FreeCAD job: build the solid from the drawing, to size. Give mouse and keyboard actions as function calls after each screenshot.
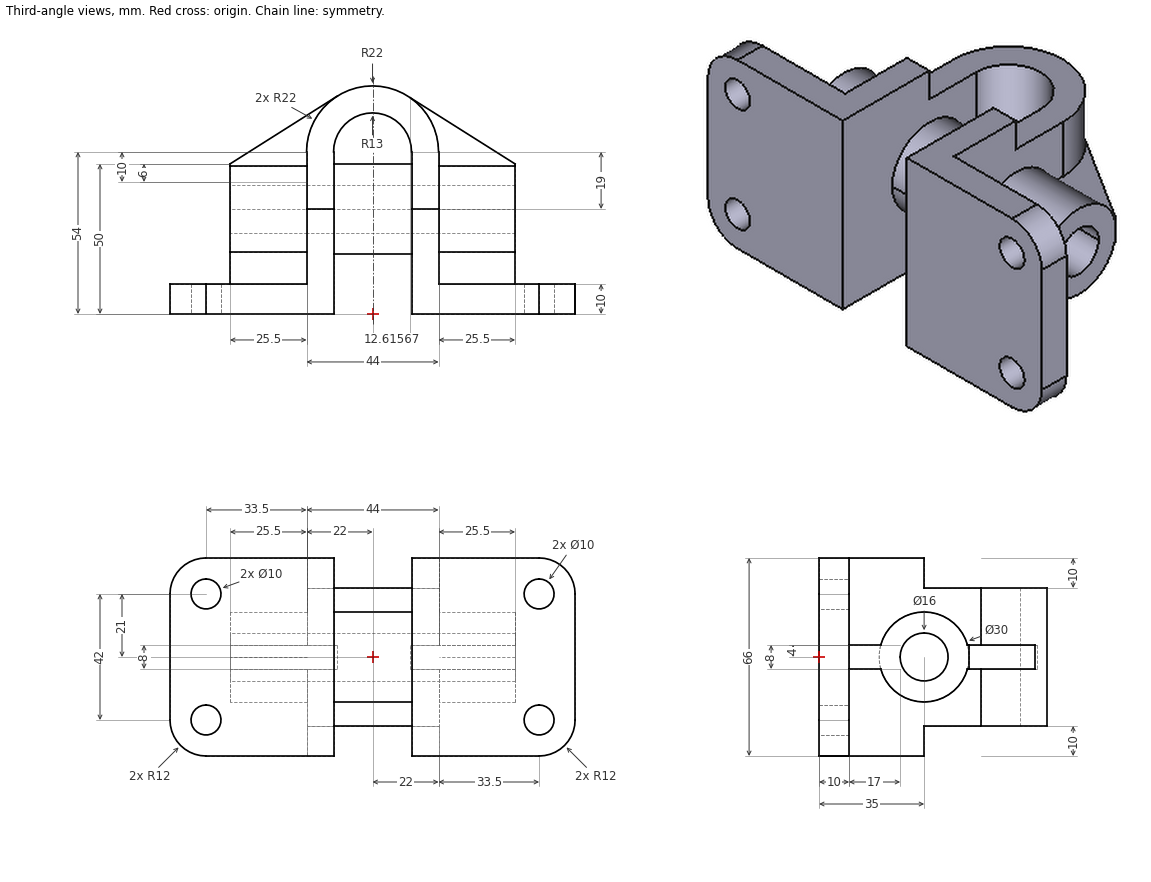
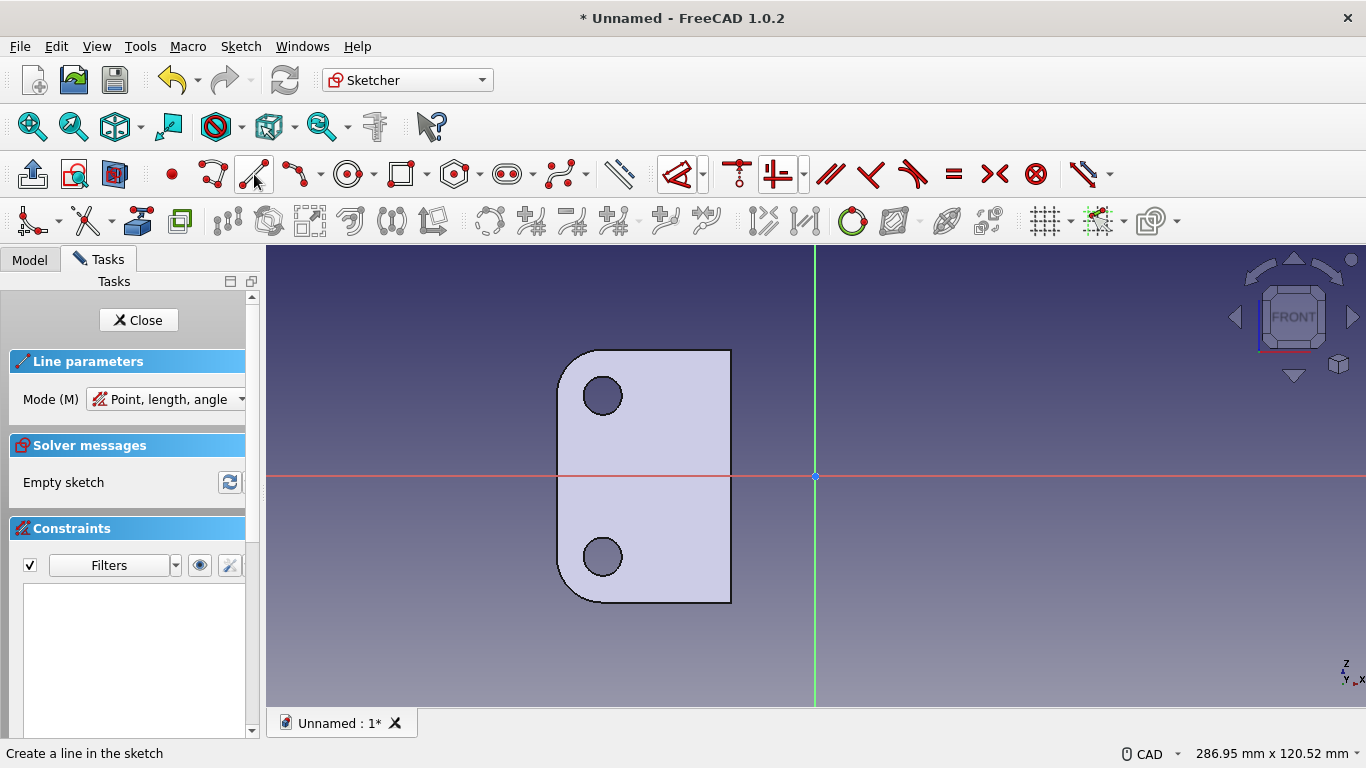
click(1074, 396)
click(1074, 557)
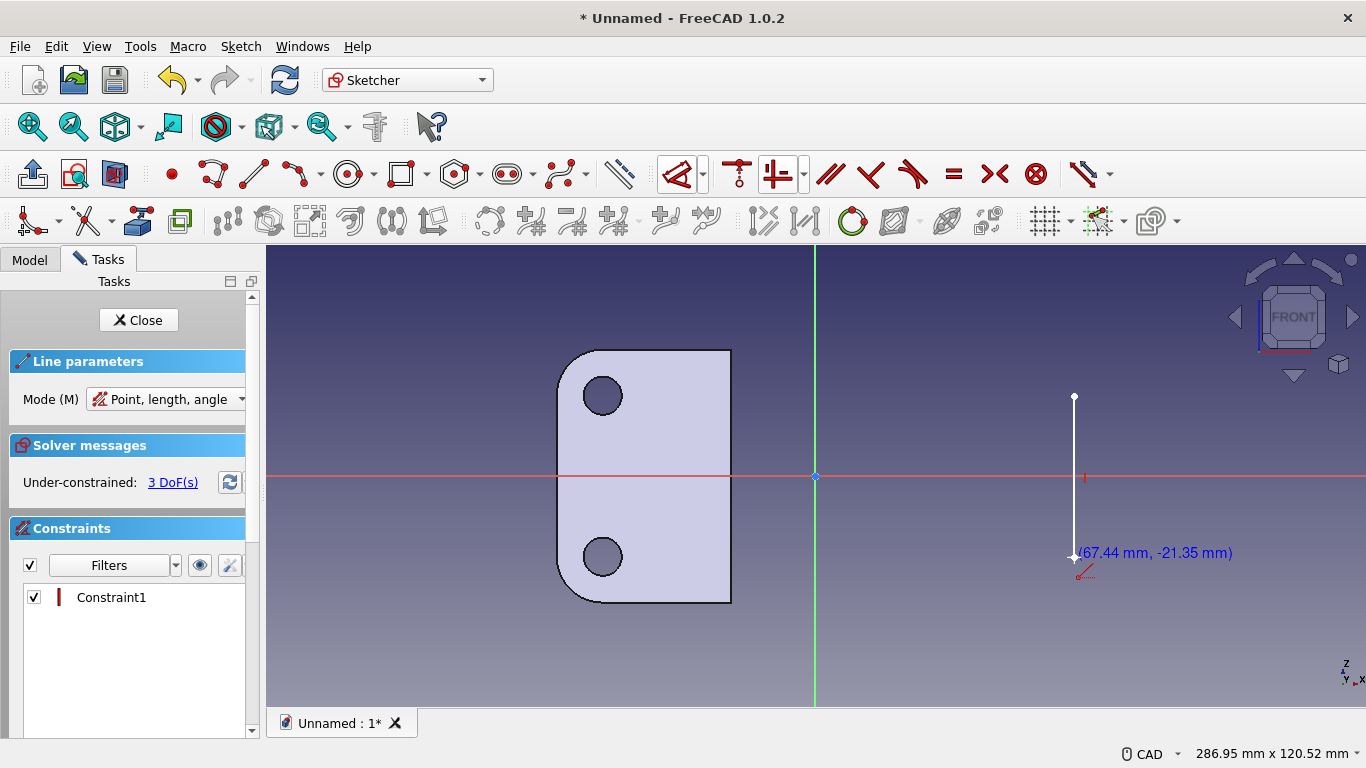
click(213, 174)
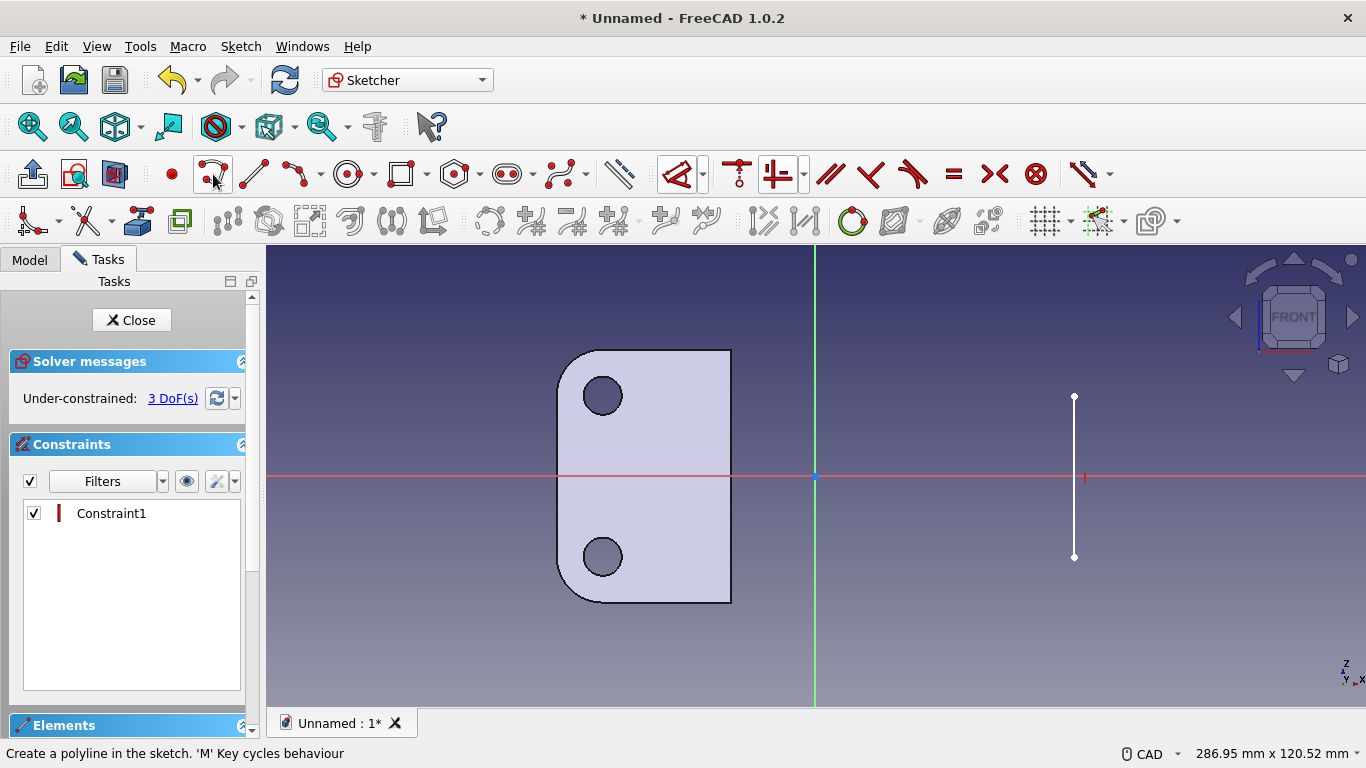
click(1028, 603)
click(900, 603)
click(900, 350)
click(1028, 350)
right_click(1028, 350)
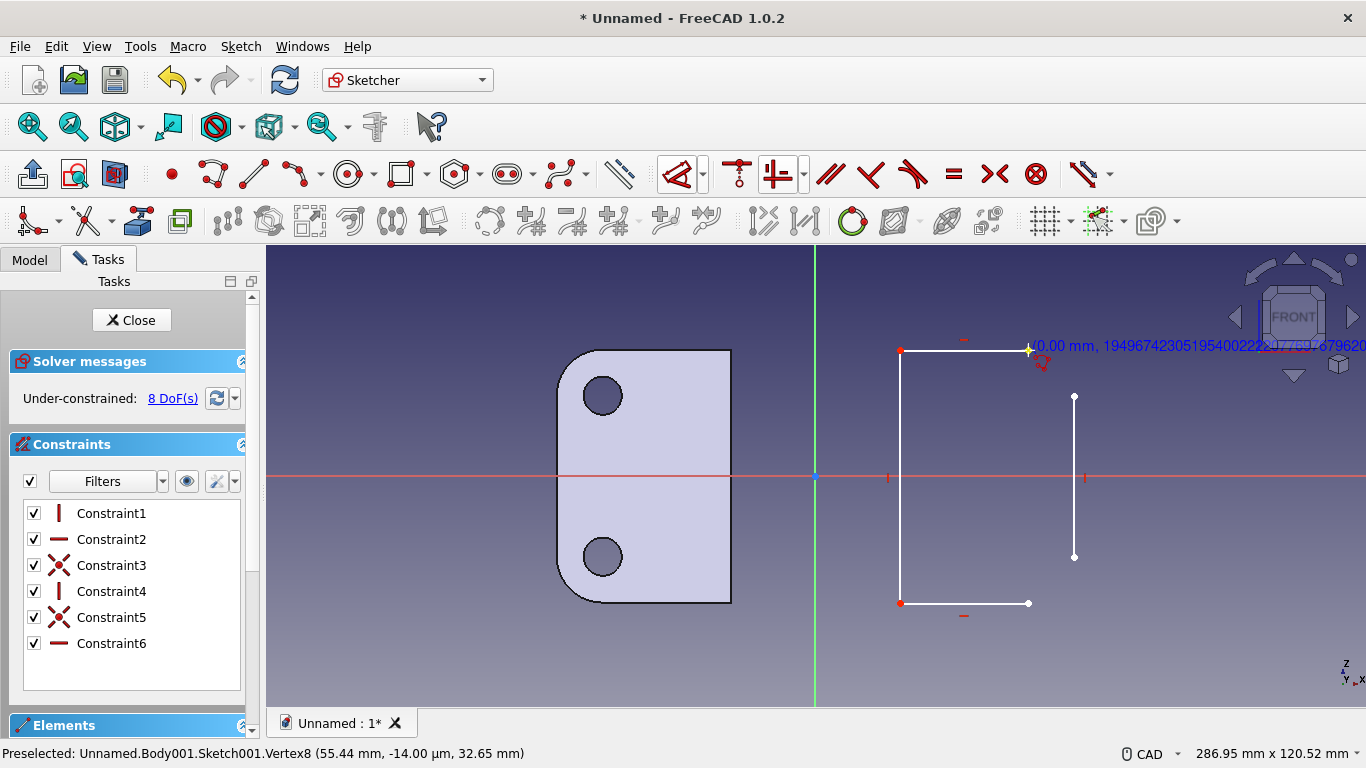
click(294, 174)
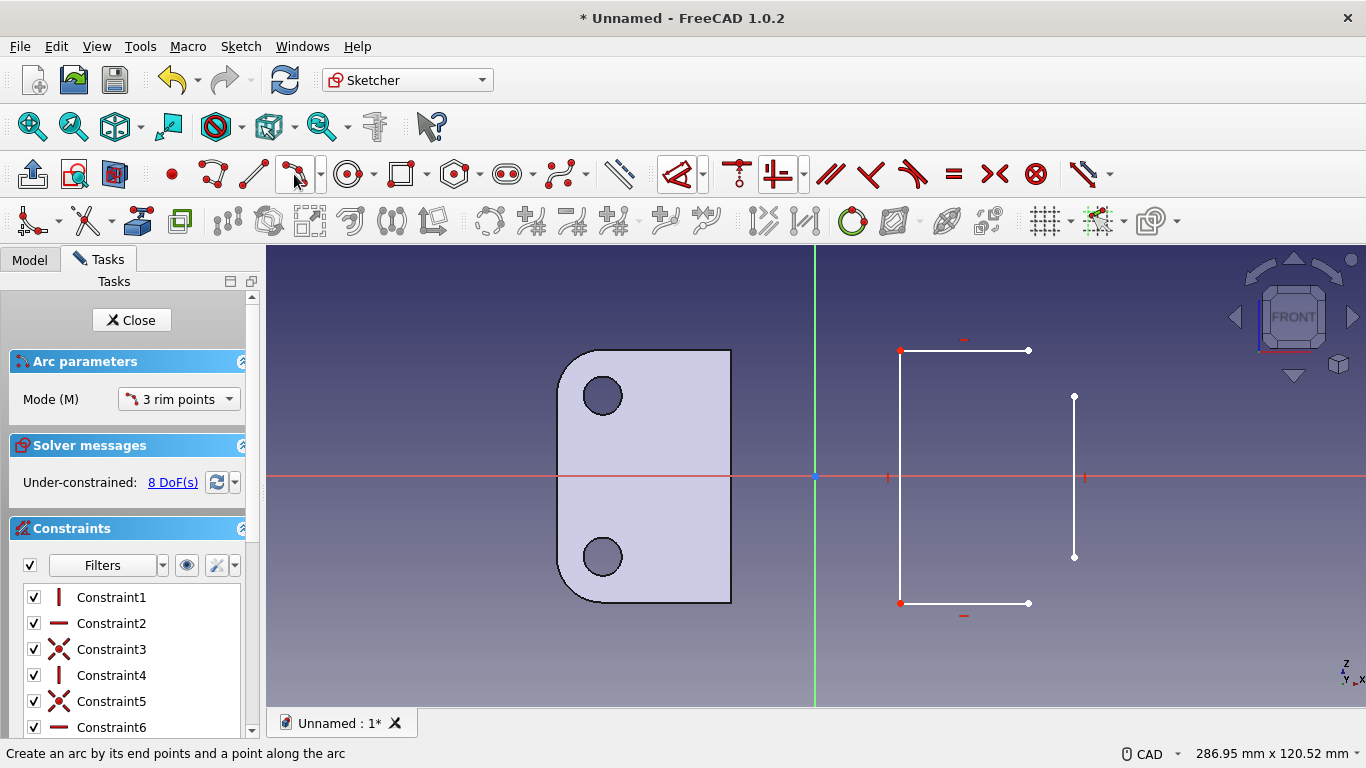
click(1074, 558)
click(1028, 604)
click(1061, 589)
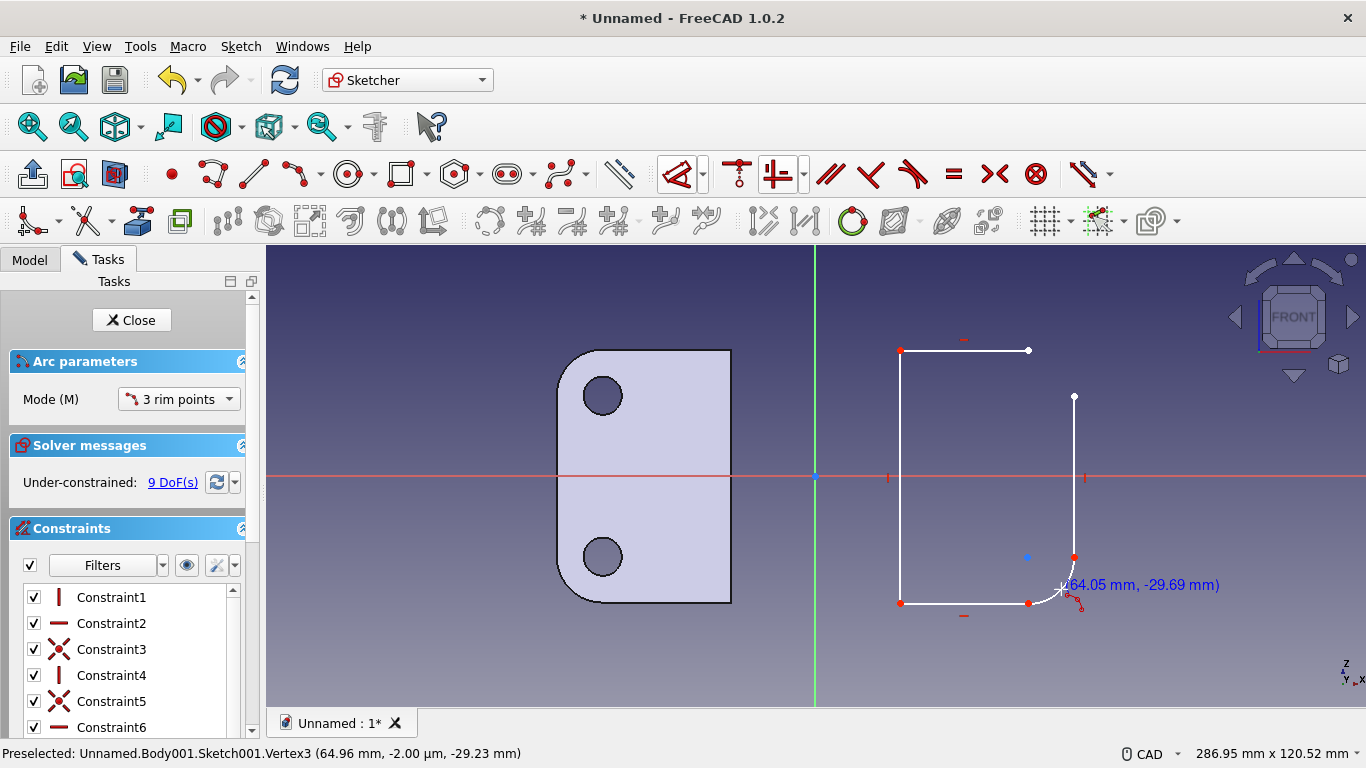
click(1028, 351)
click(1074, 397)
click(1061, 363)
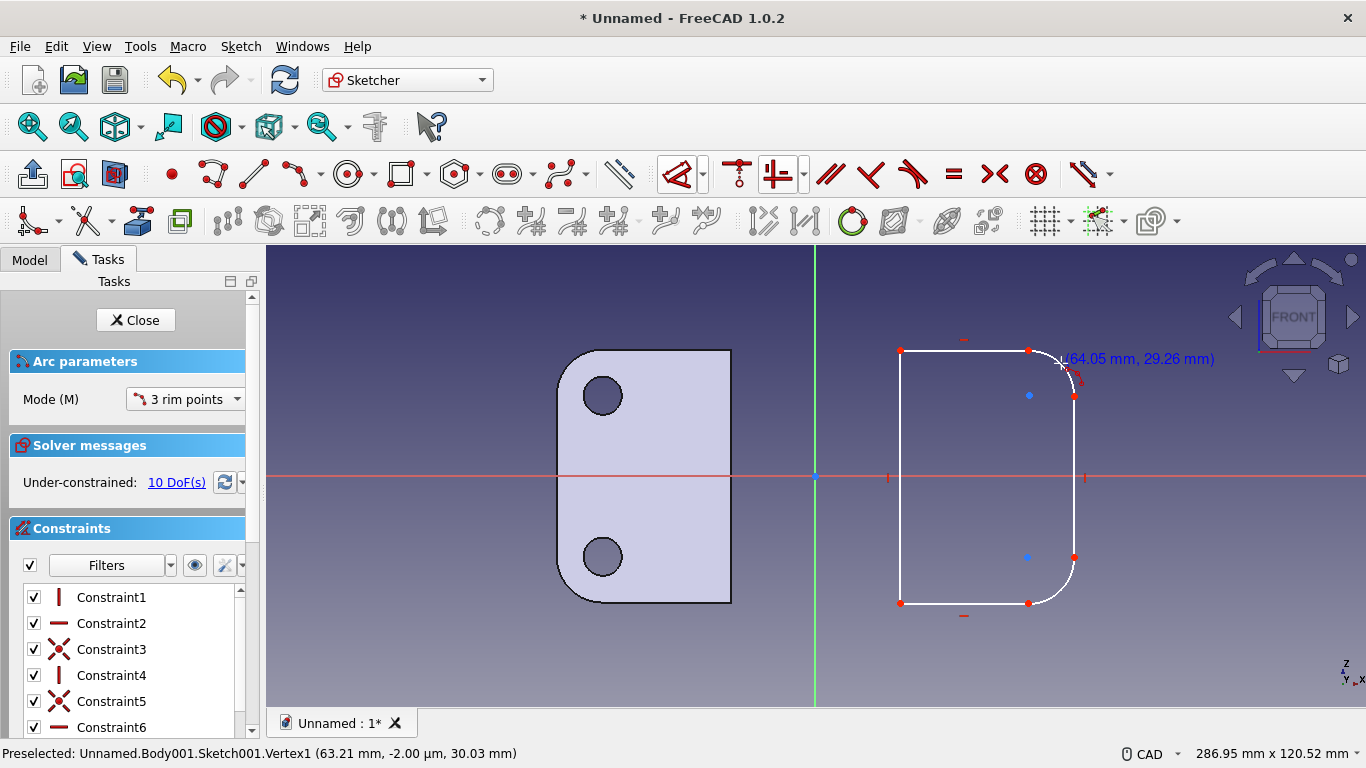
click(348, 174)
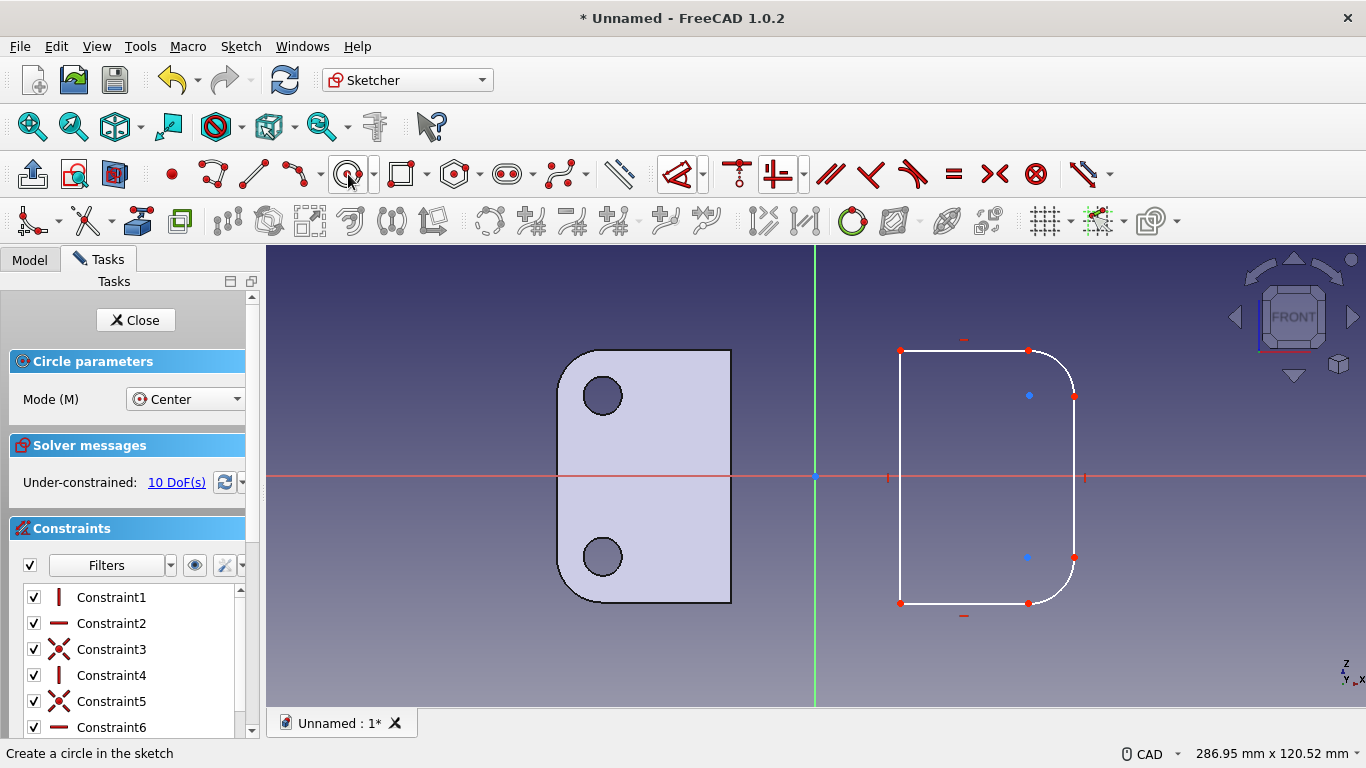
click(1028, 396)
move(1042, 382)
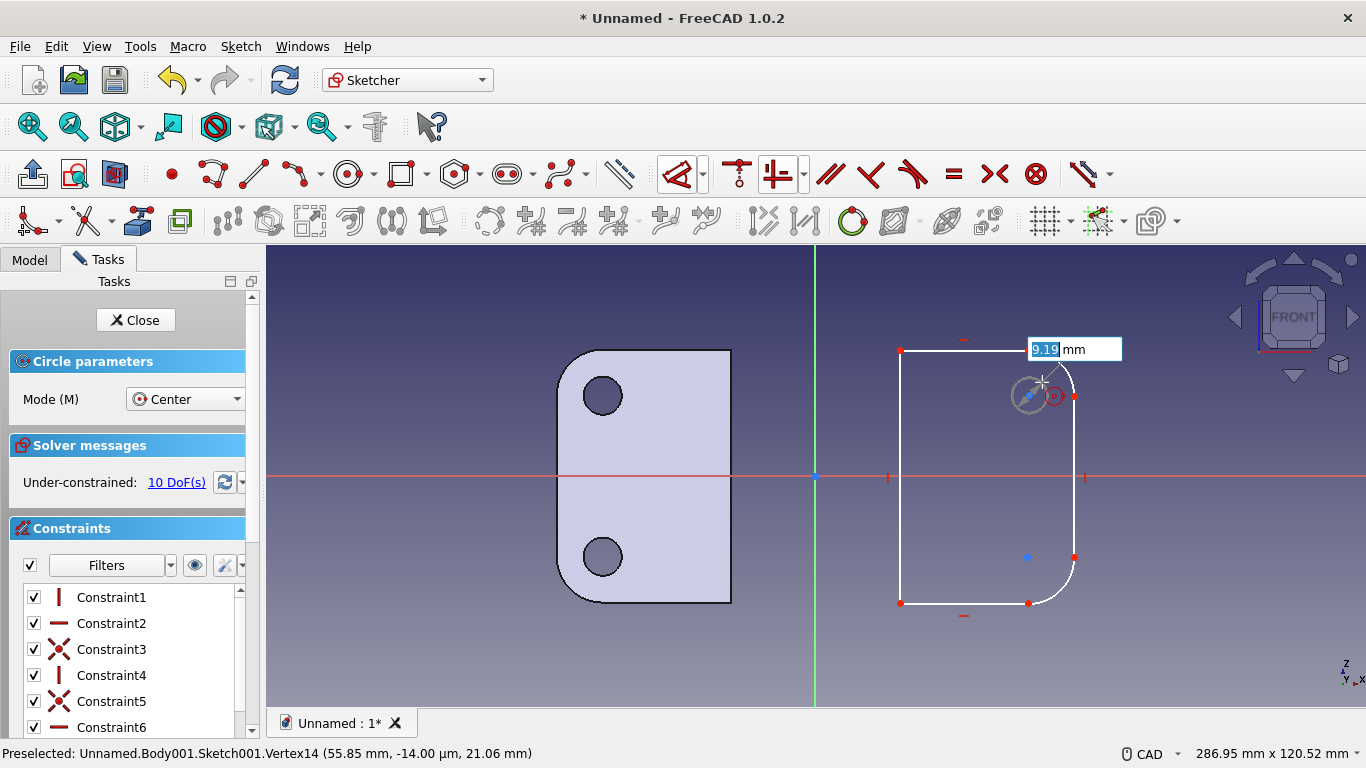
text(10)
key(Return)